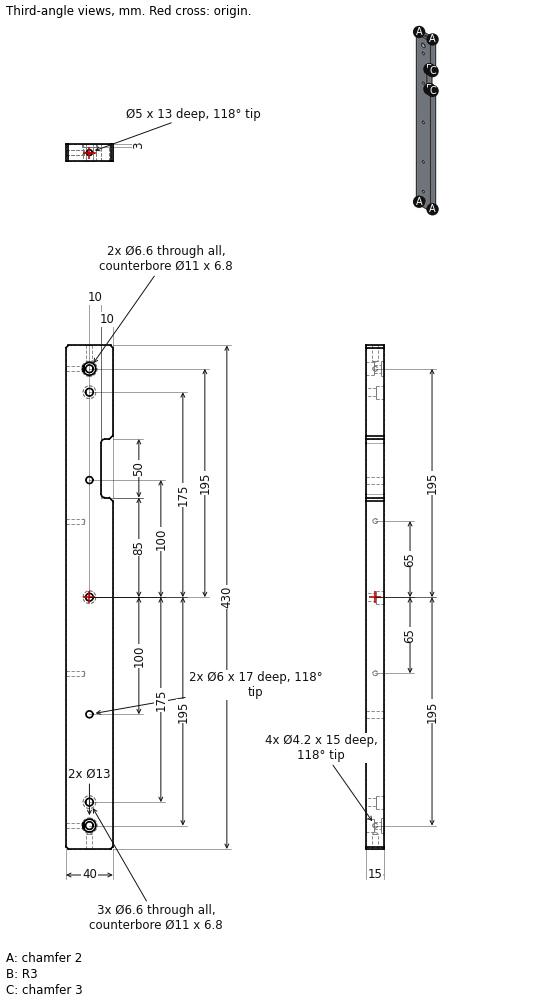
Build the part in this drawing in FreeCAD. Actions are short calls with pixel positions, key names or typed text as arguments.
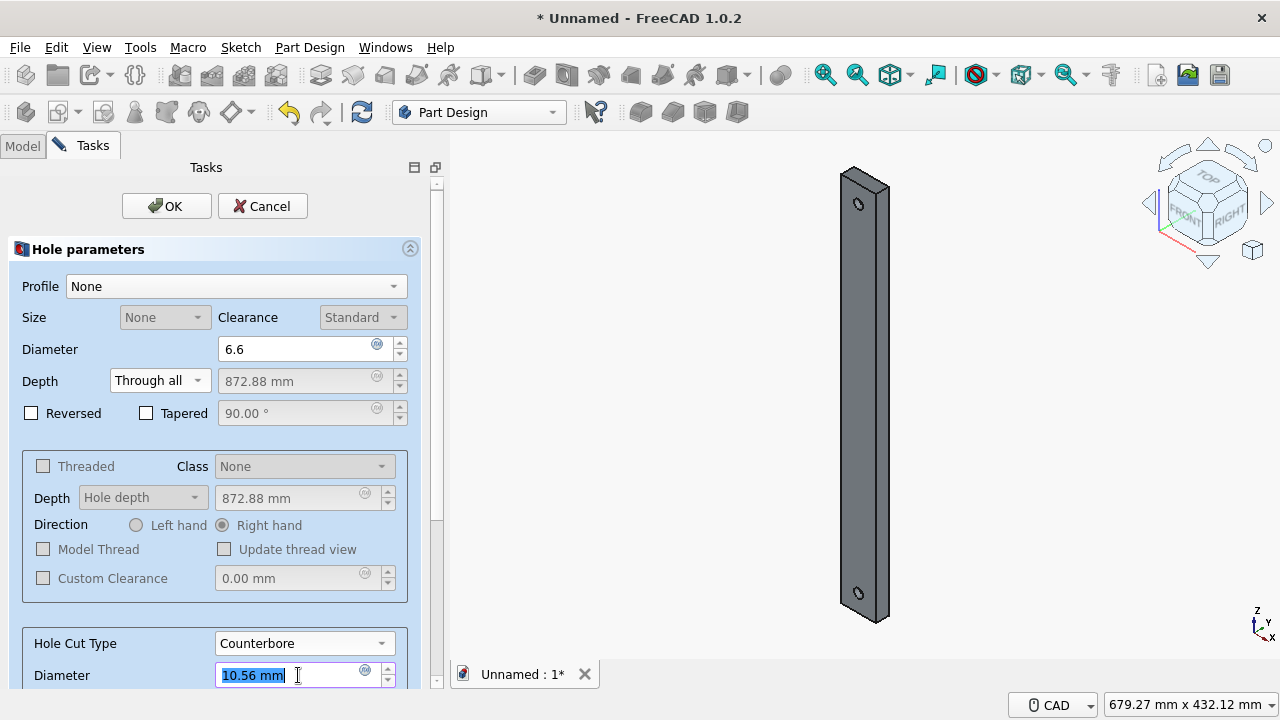
text(11)
key(Tab)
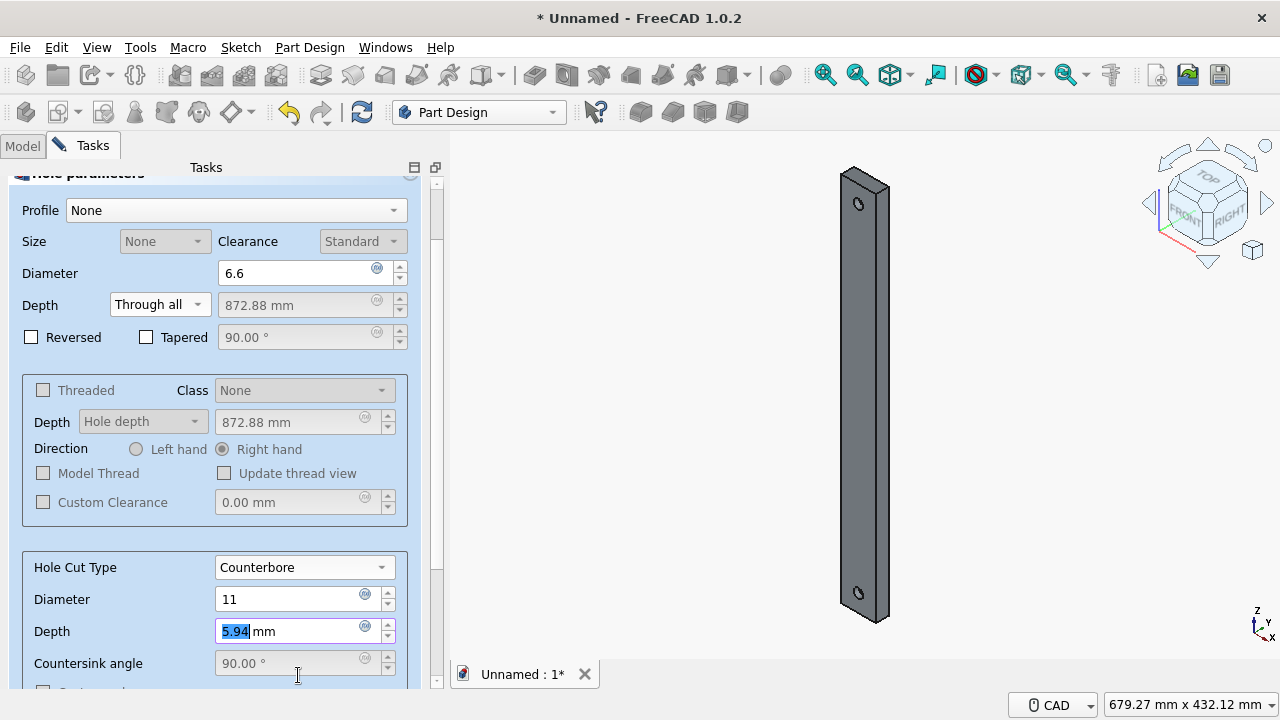
text(6.8)
key(Tab)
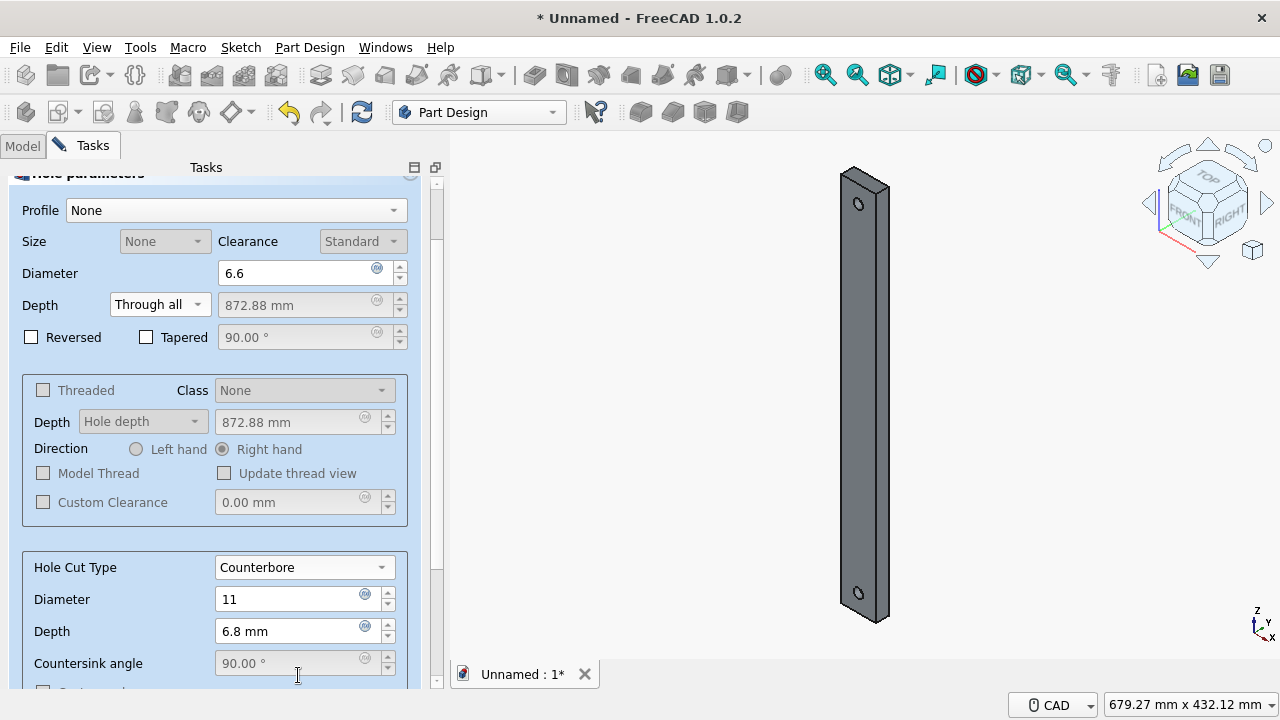
scroll(437, 432, up, 3)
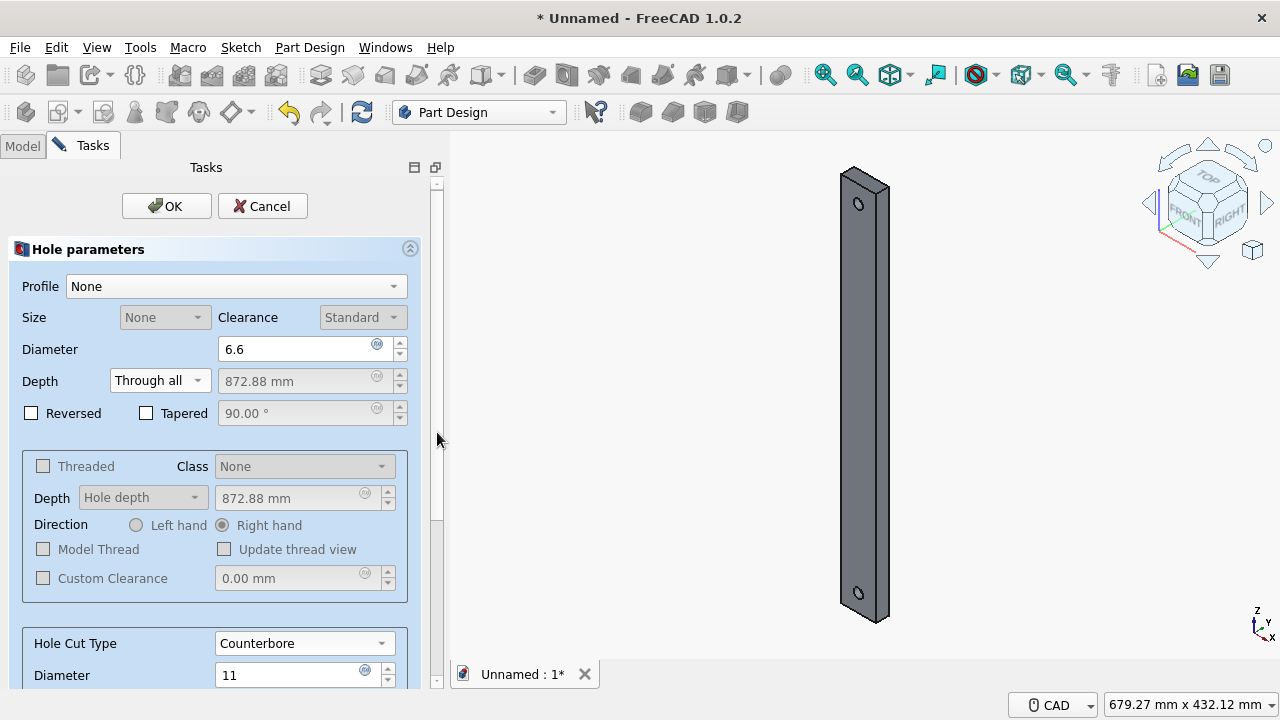
click(167, 206)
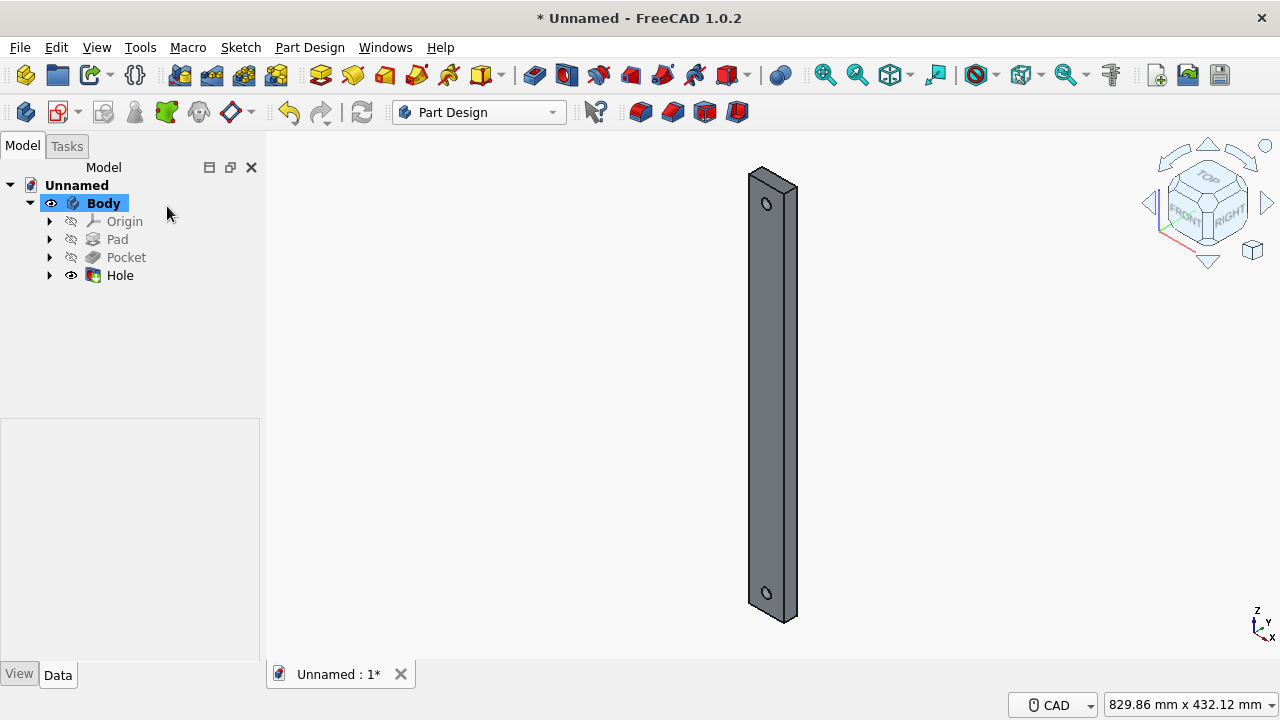
key(6)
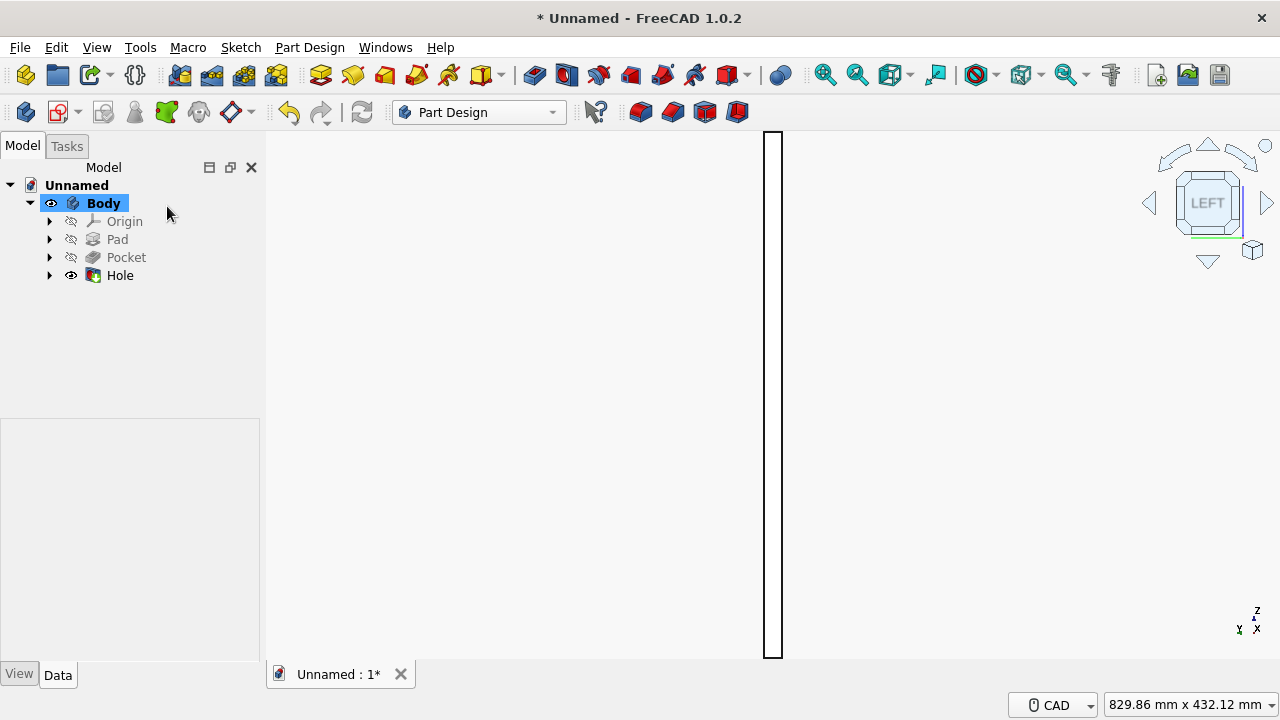
click(773, 244)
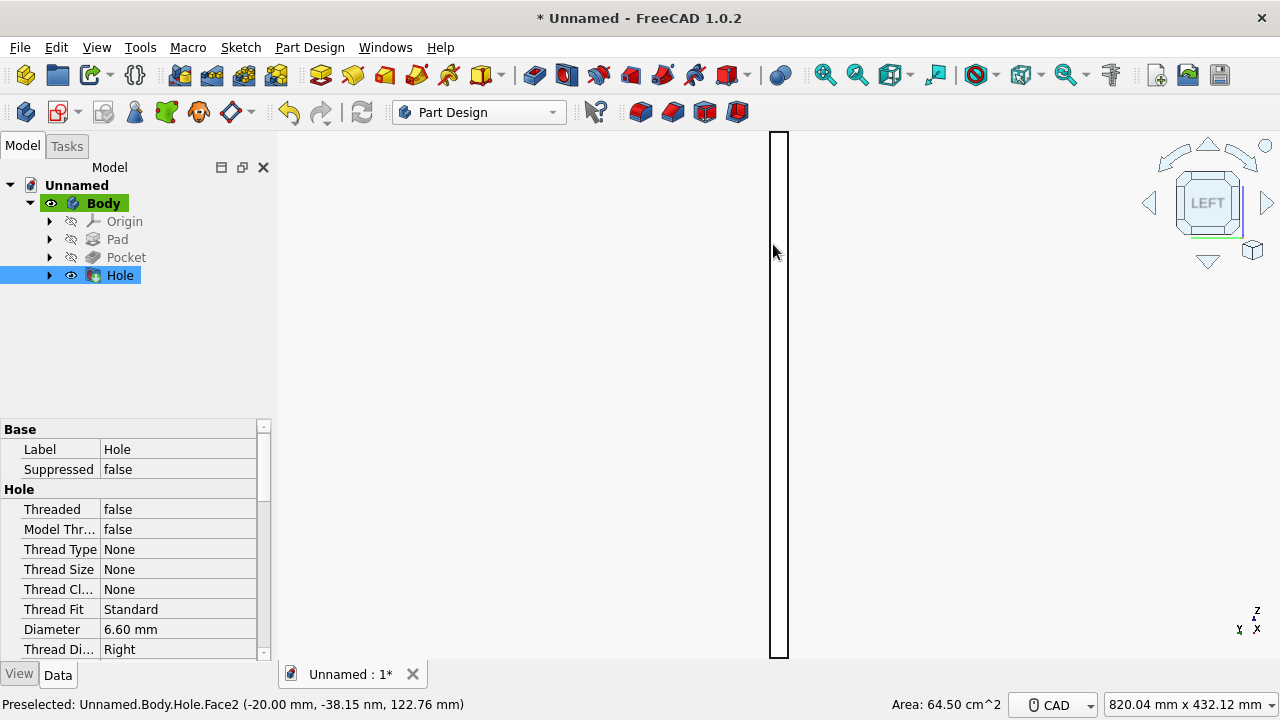
click(58, 112)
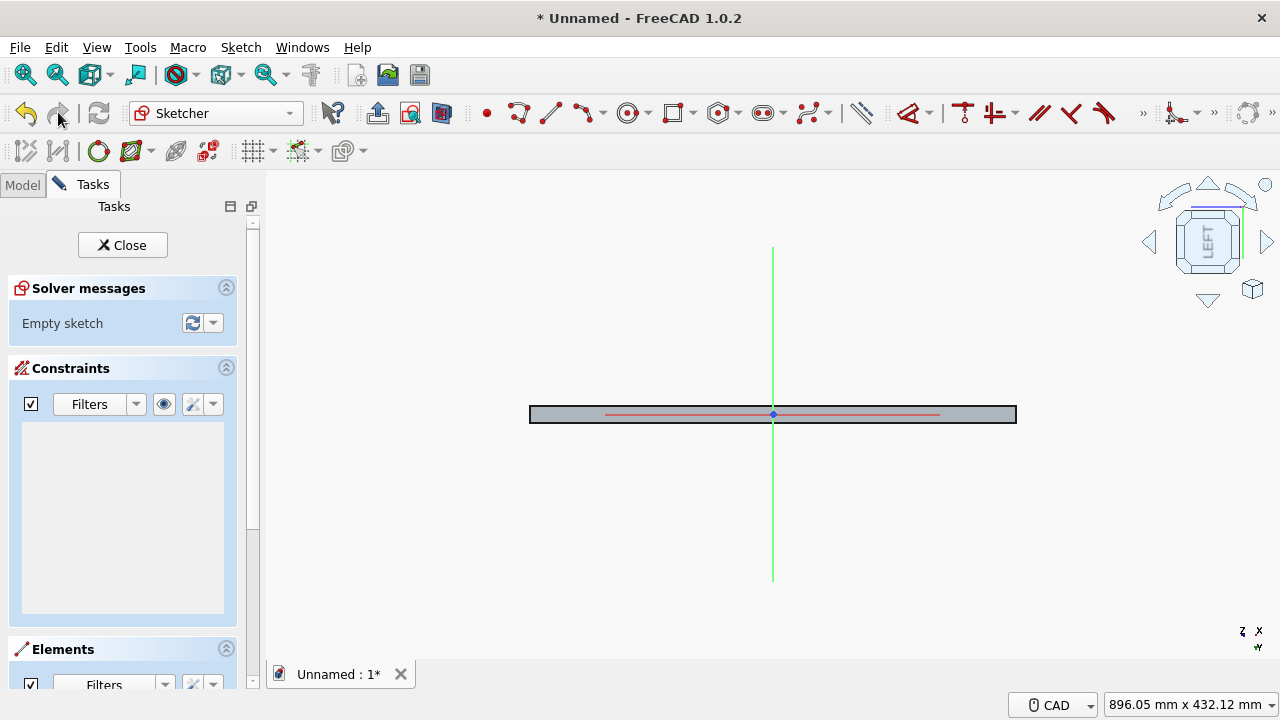
click(628, 114)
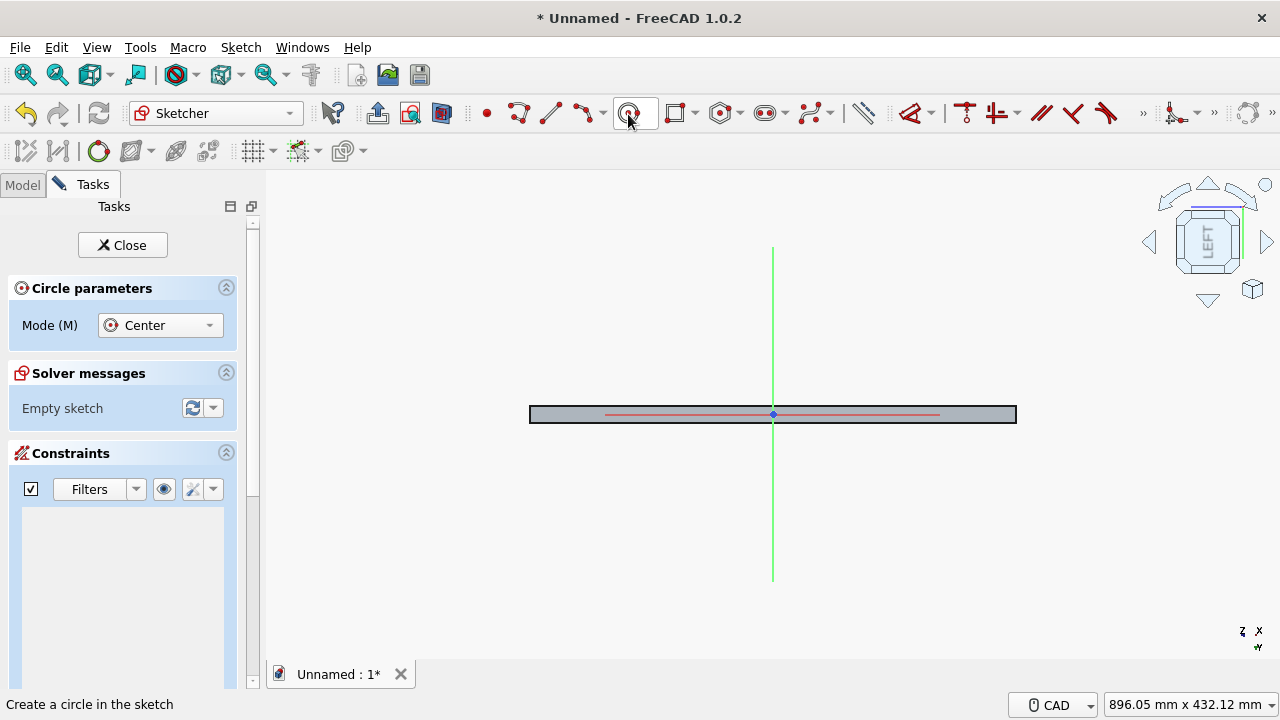
scroll(994, 415, up, 12)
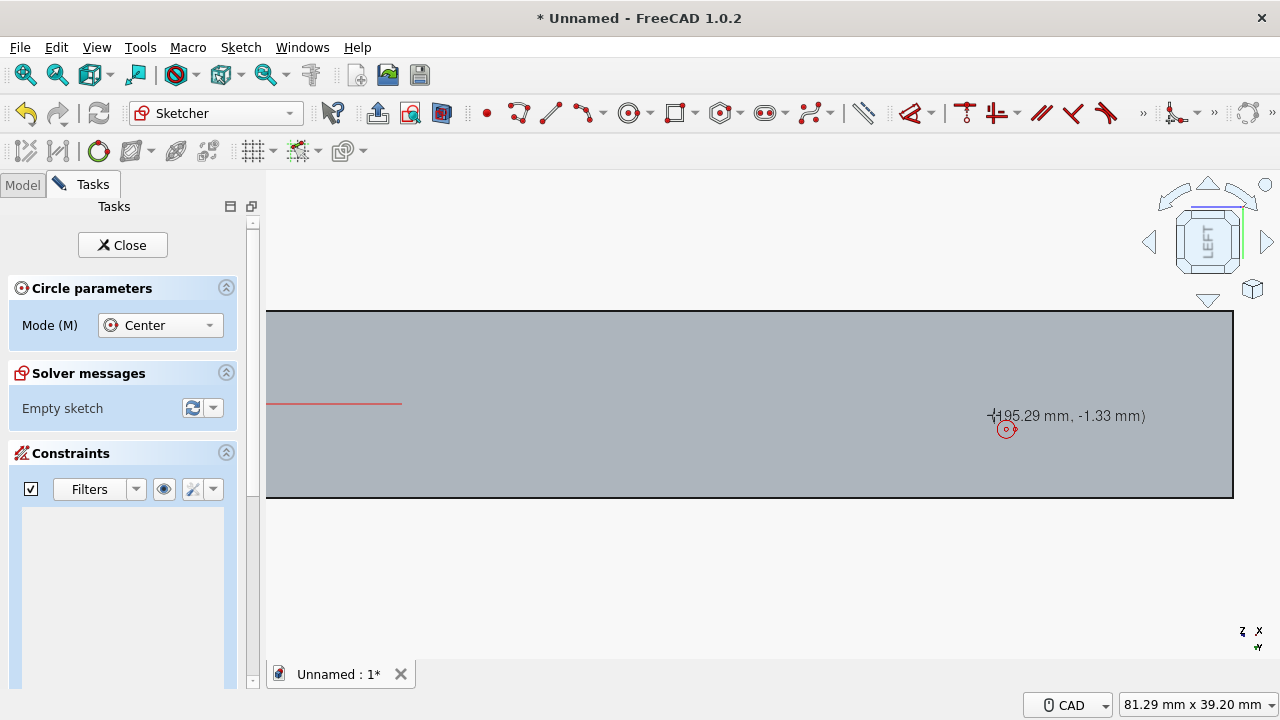
scroll(973, 416, down, 11)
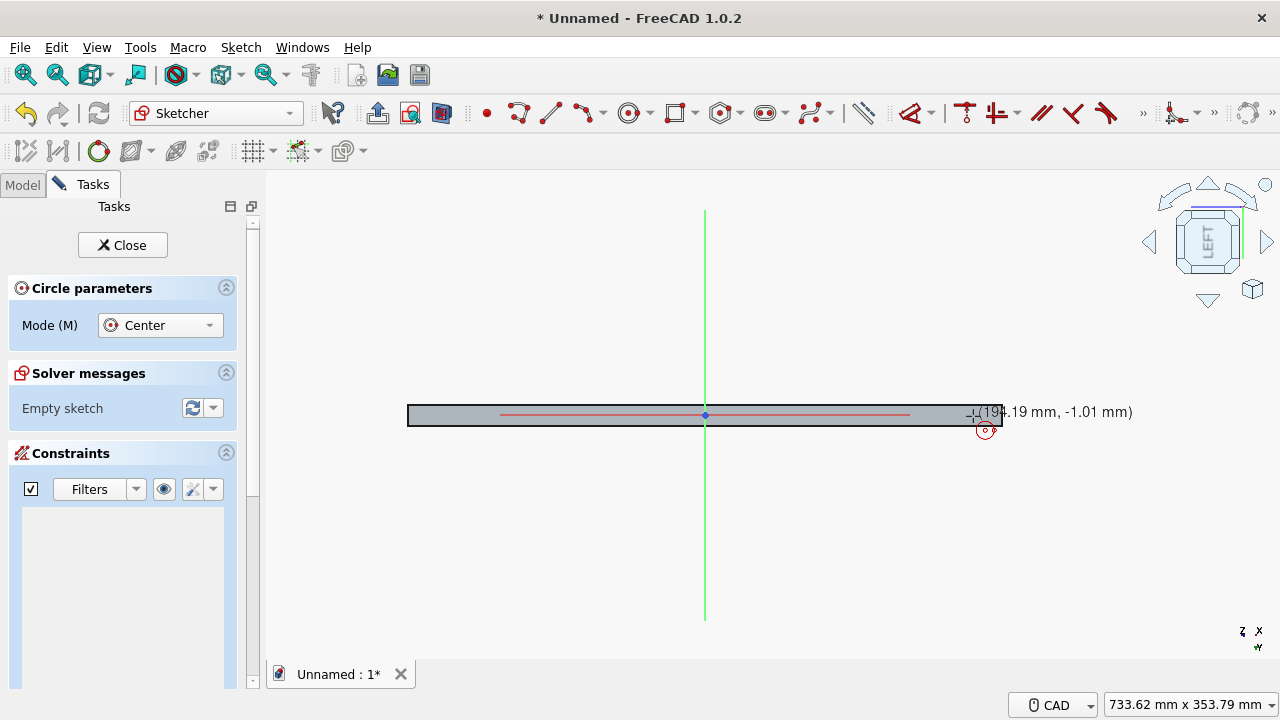
click(975, 415)